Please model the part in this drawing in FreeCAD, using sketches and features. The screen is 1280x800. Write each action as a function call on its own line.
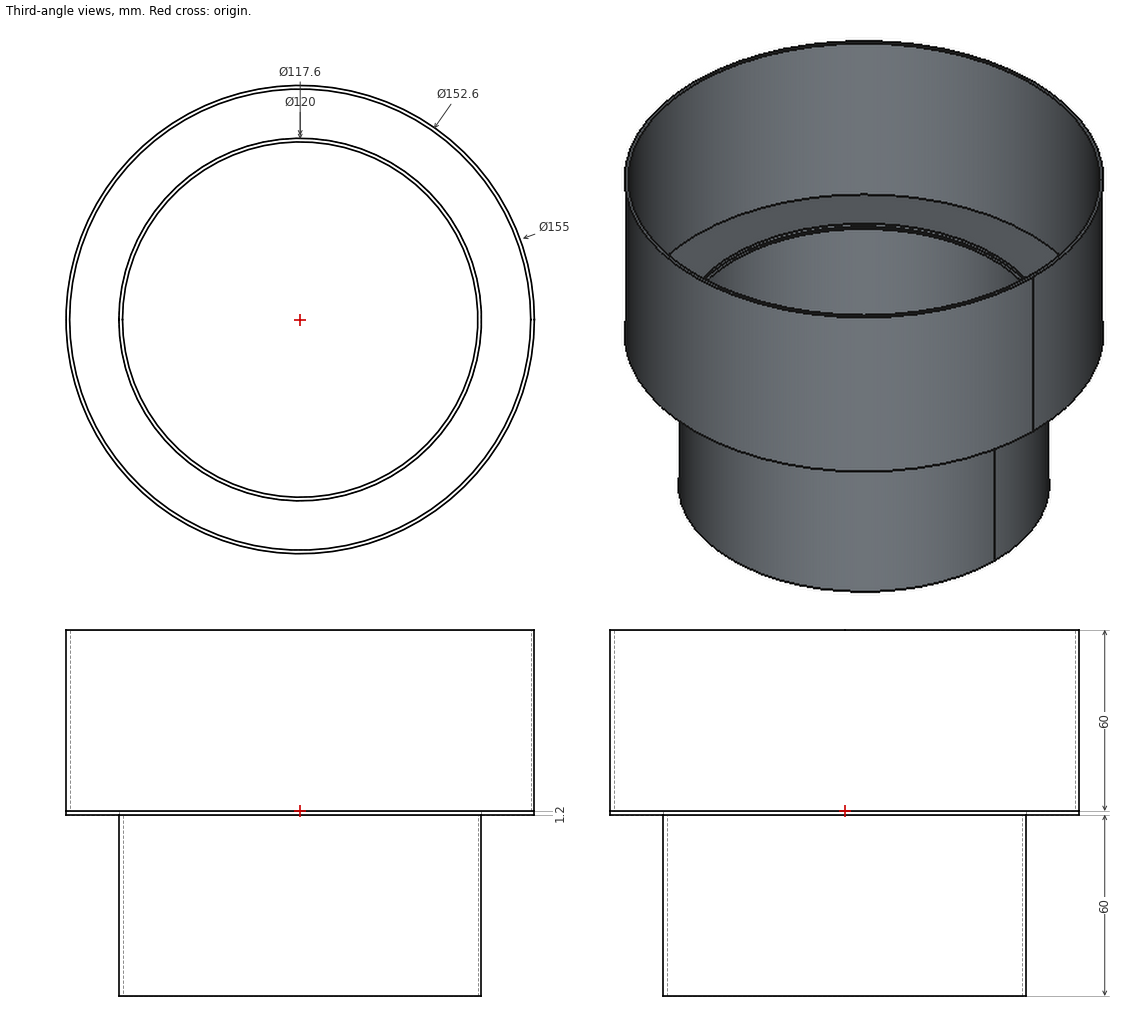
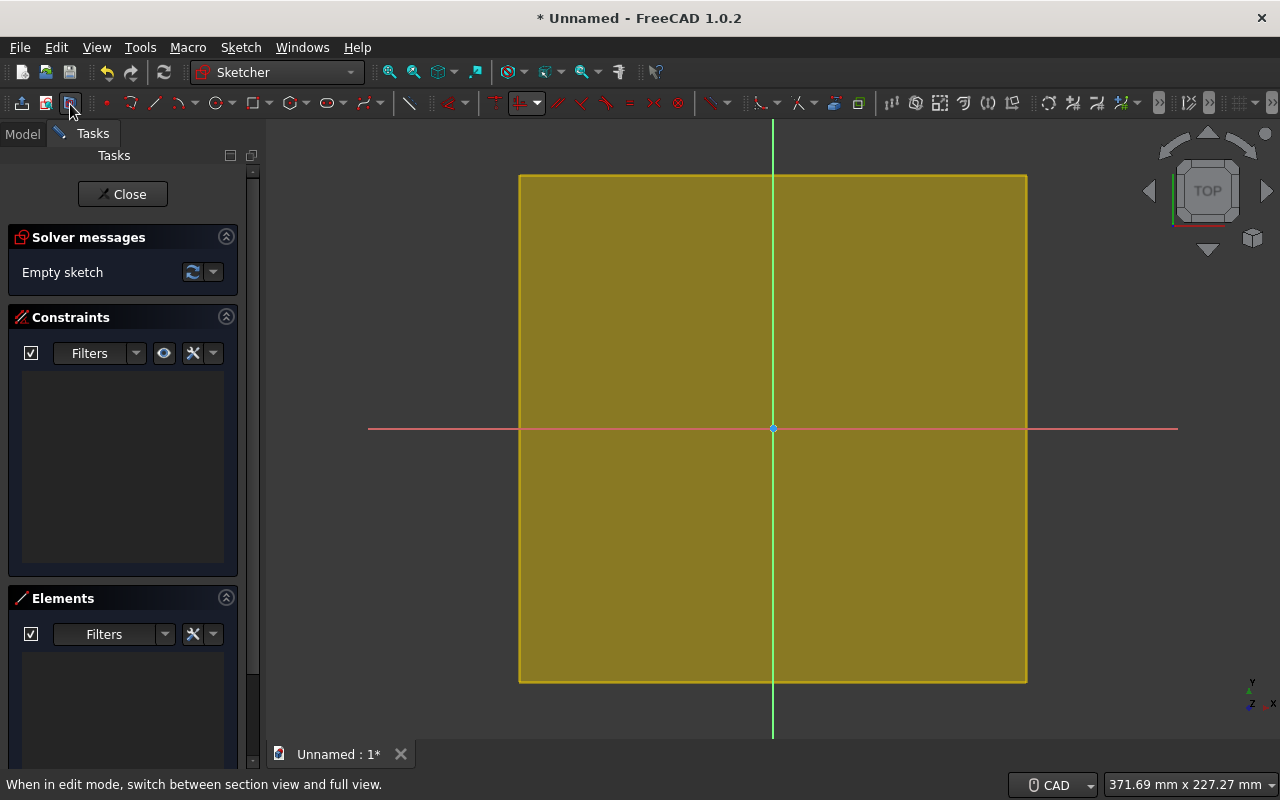
click(216, 104)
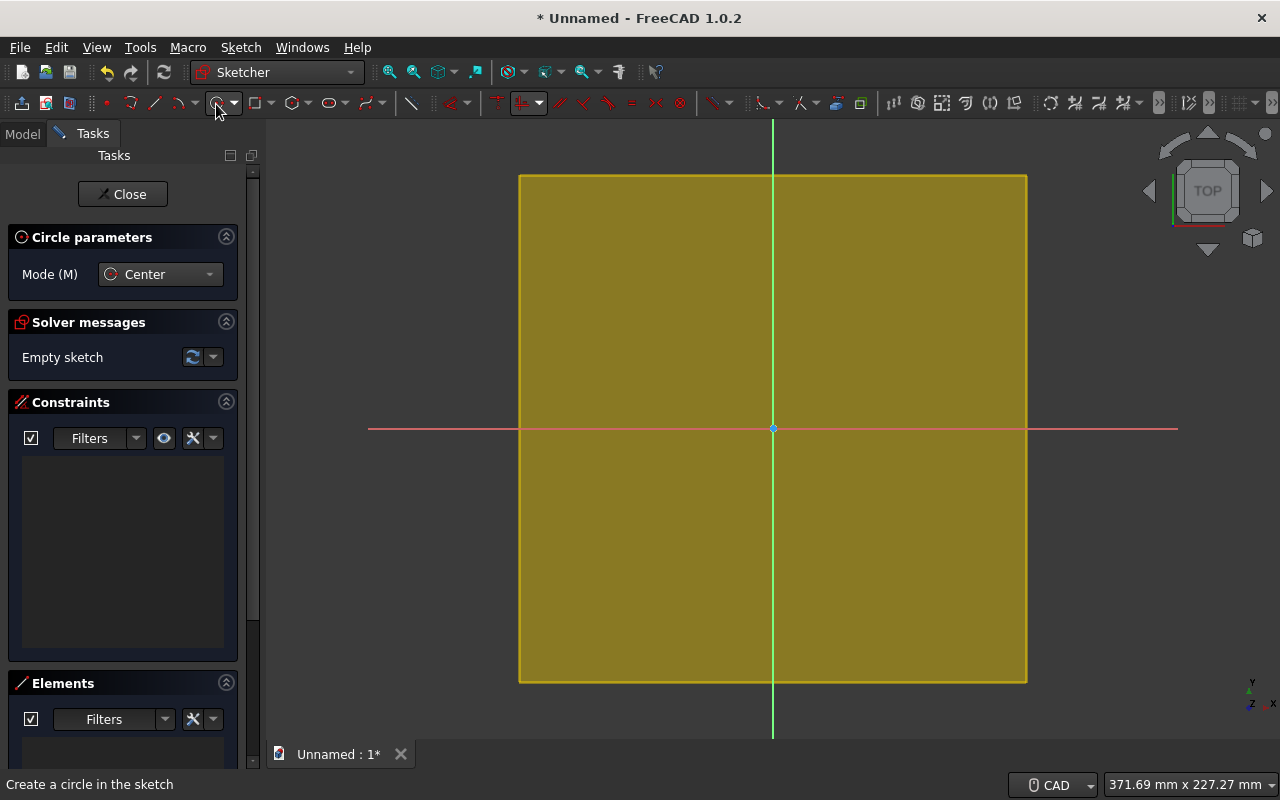
click(773, 429)
click(923, 279)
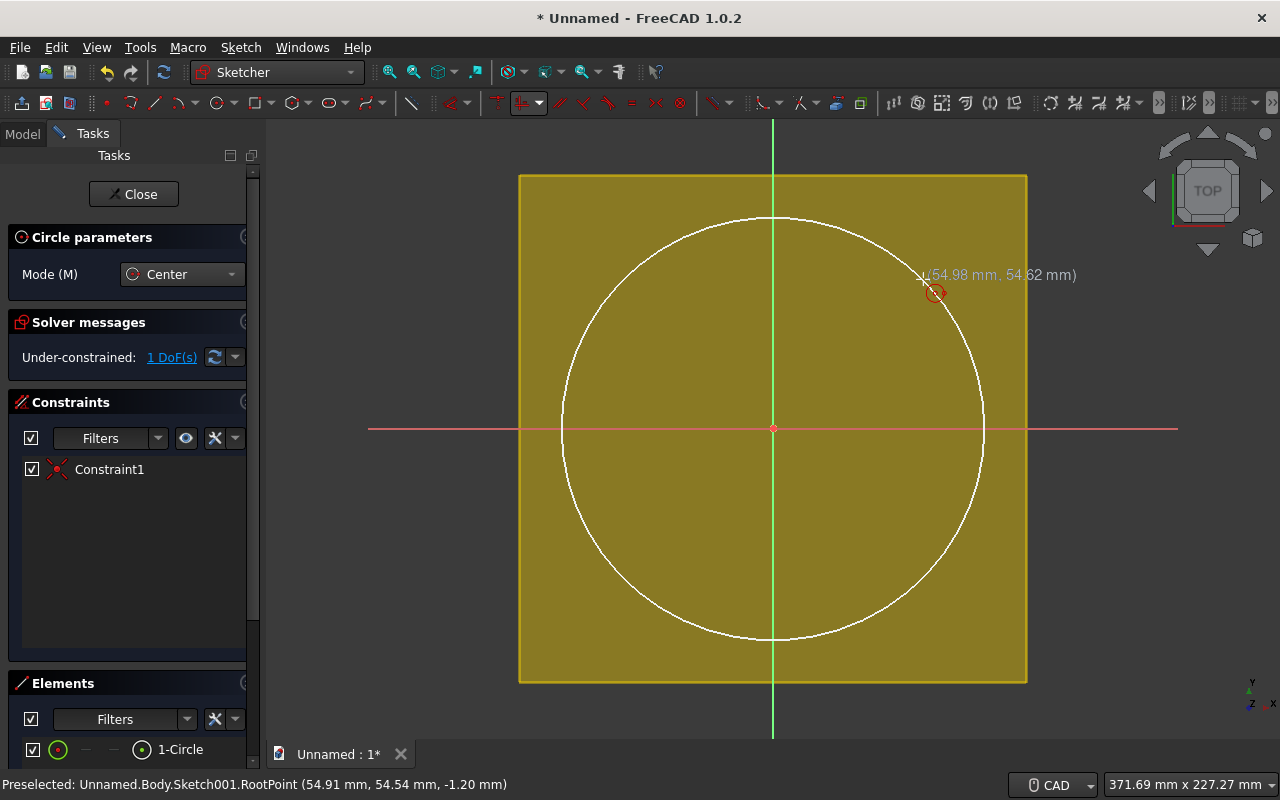
click(773, 429)
click(889, 313)
key(Escape)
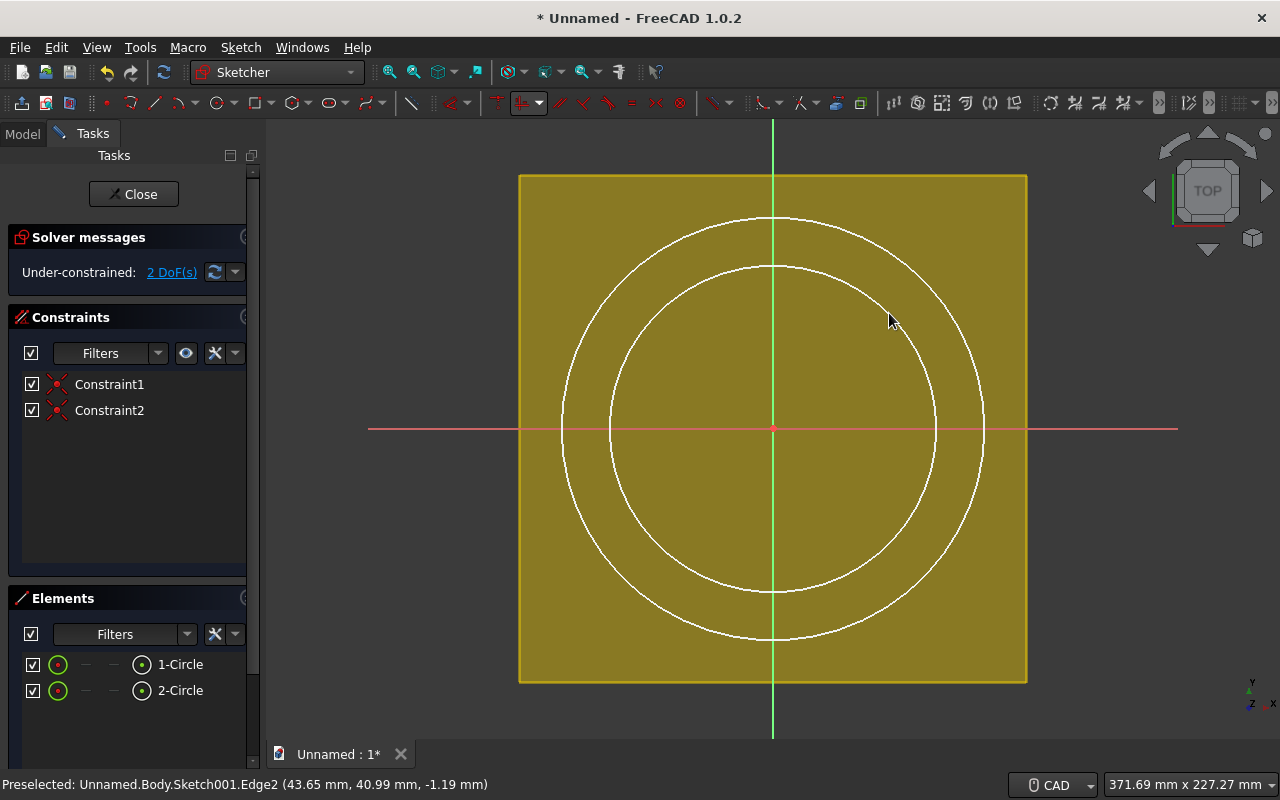
click(450, 104)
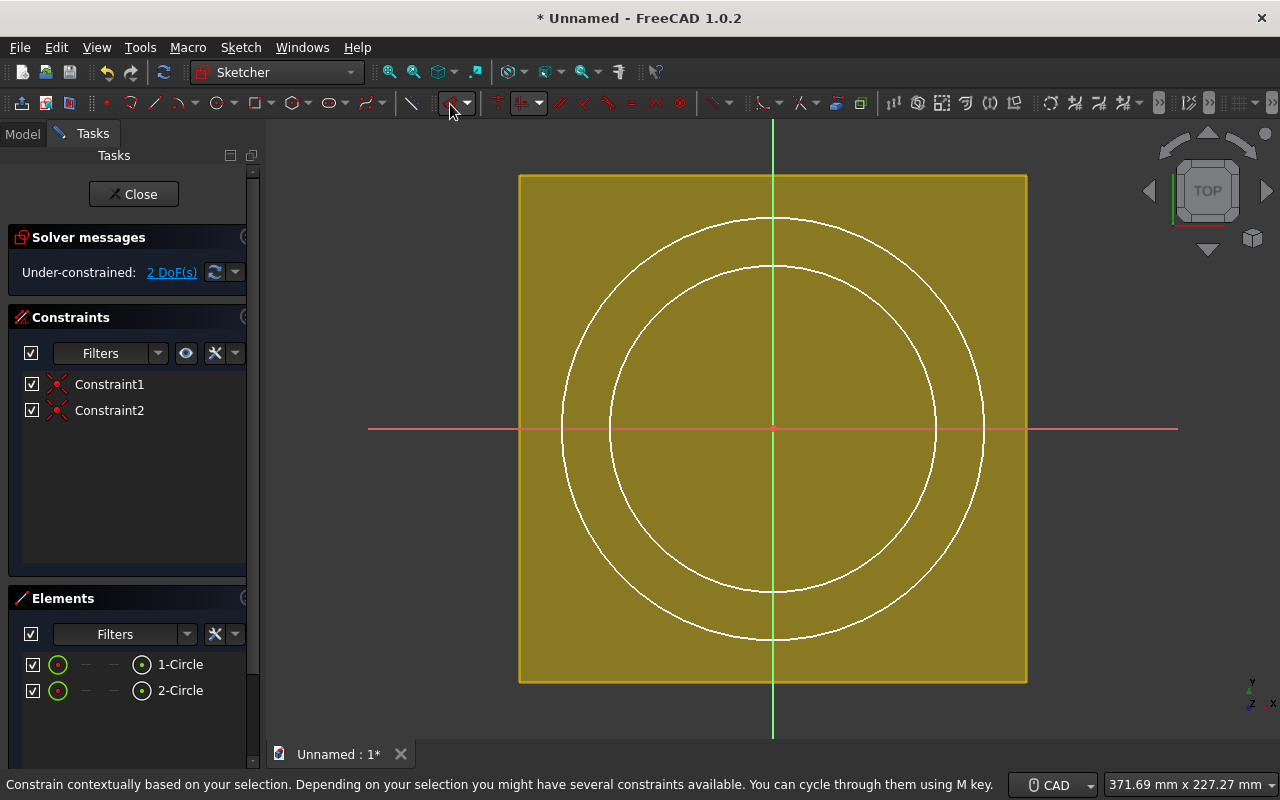
click(922, 279)
click(945, 256)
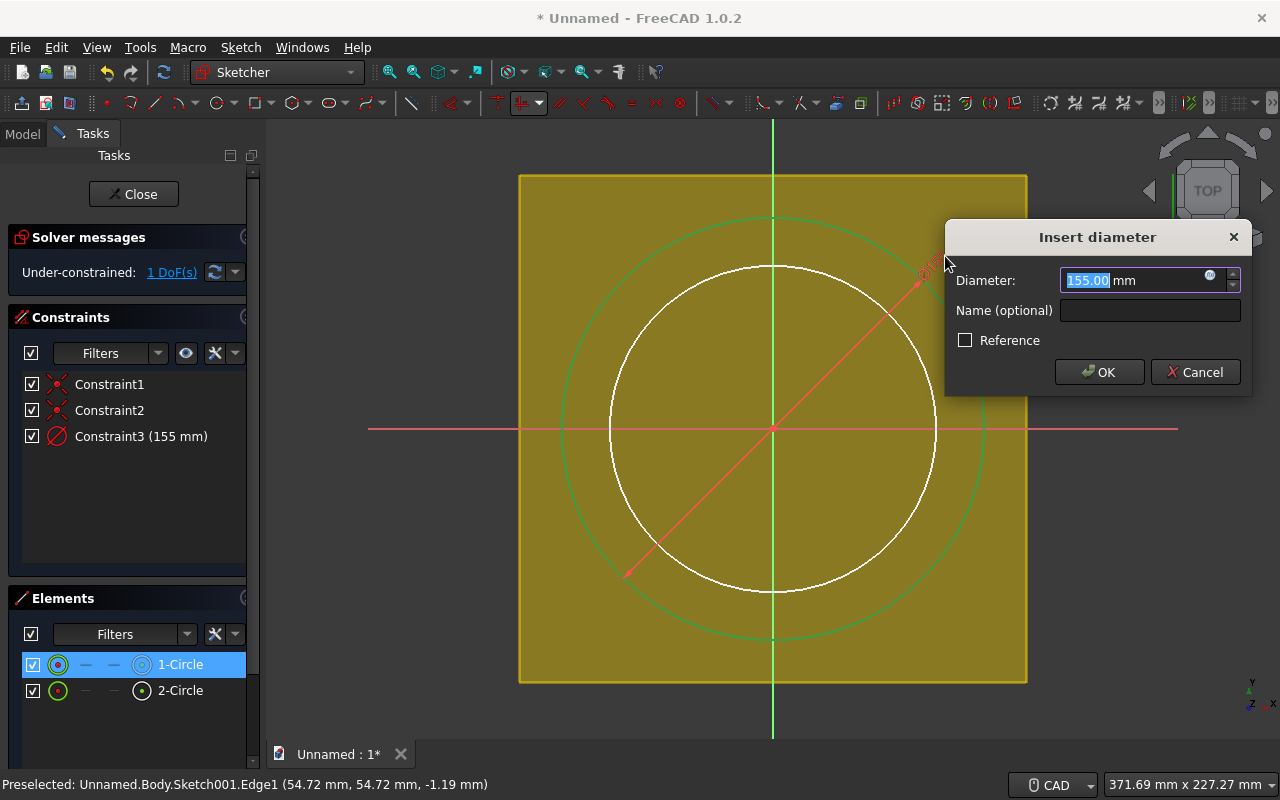
text(155)
key(Return)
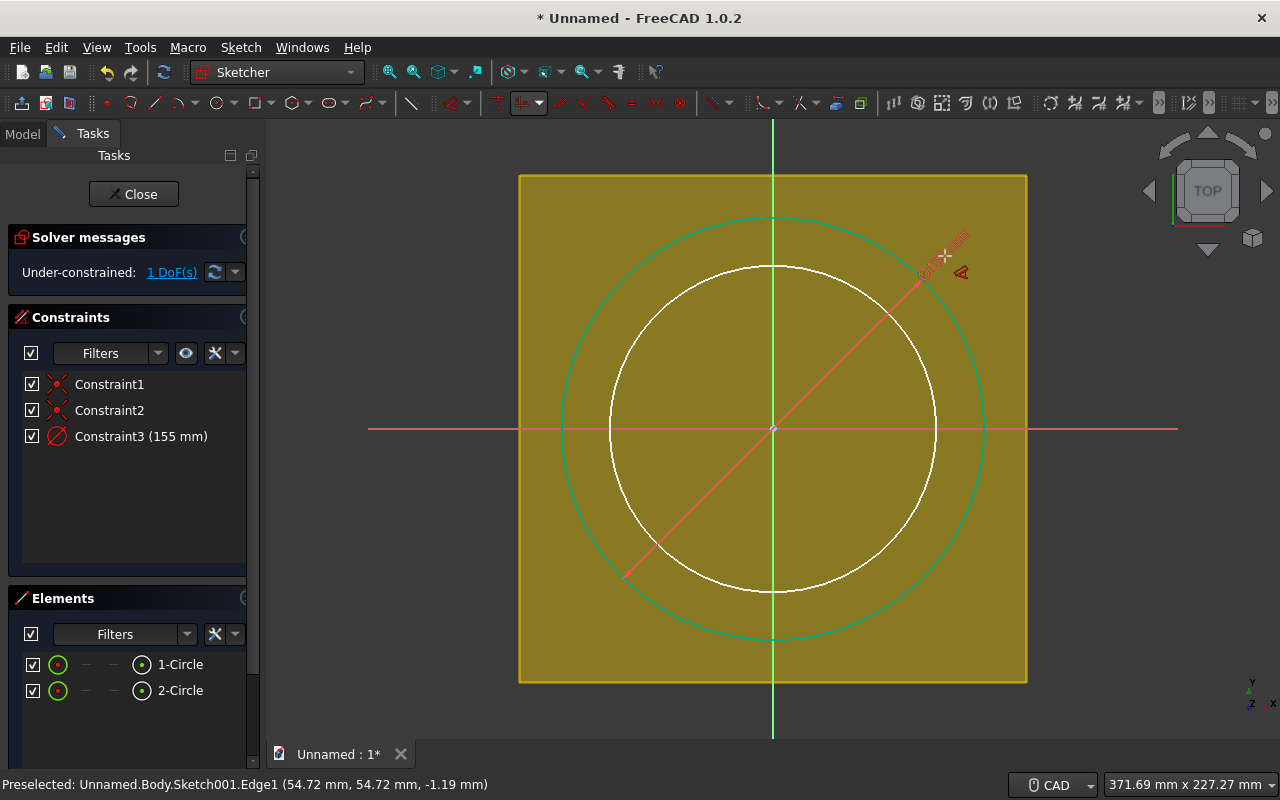
click(888, 313)
click(911, 290)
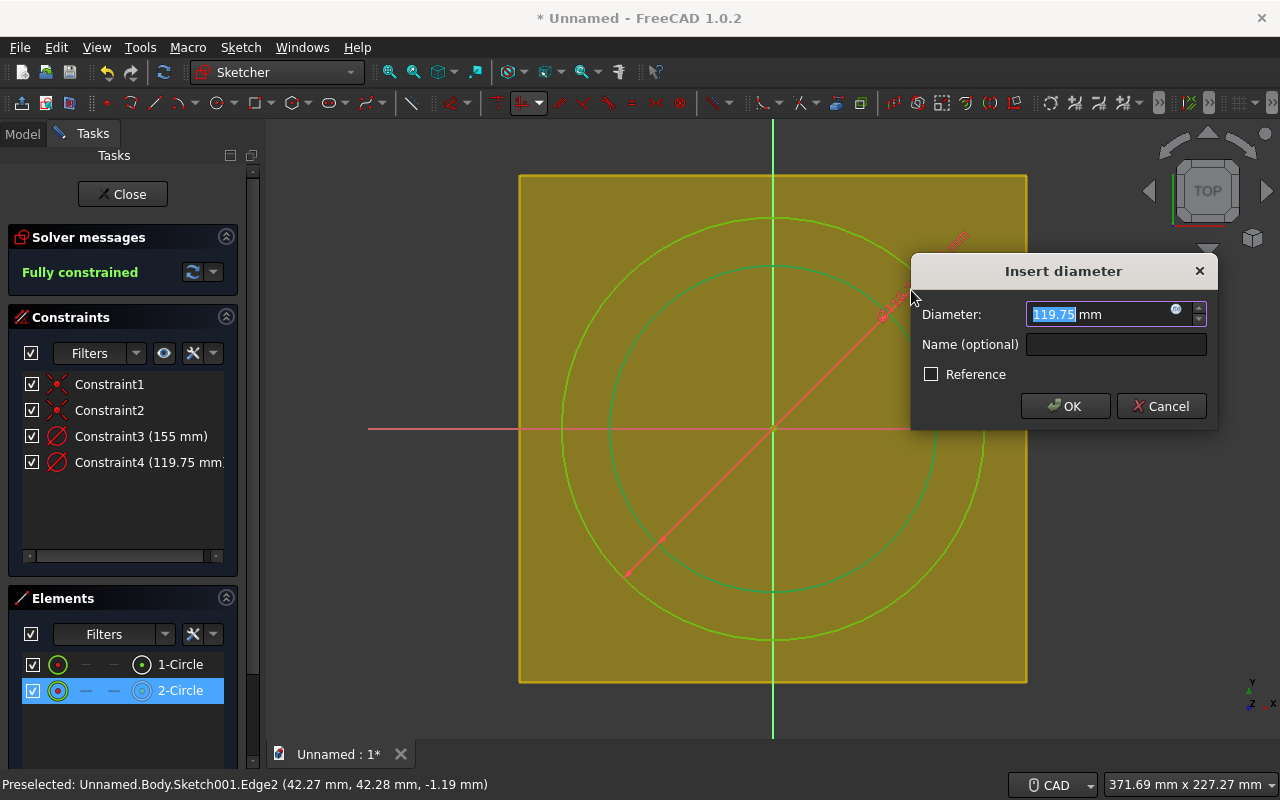
text(120)
key(Return)
key(Escape)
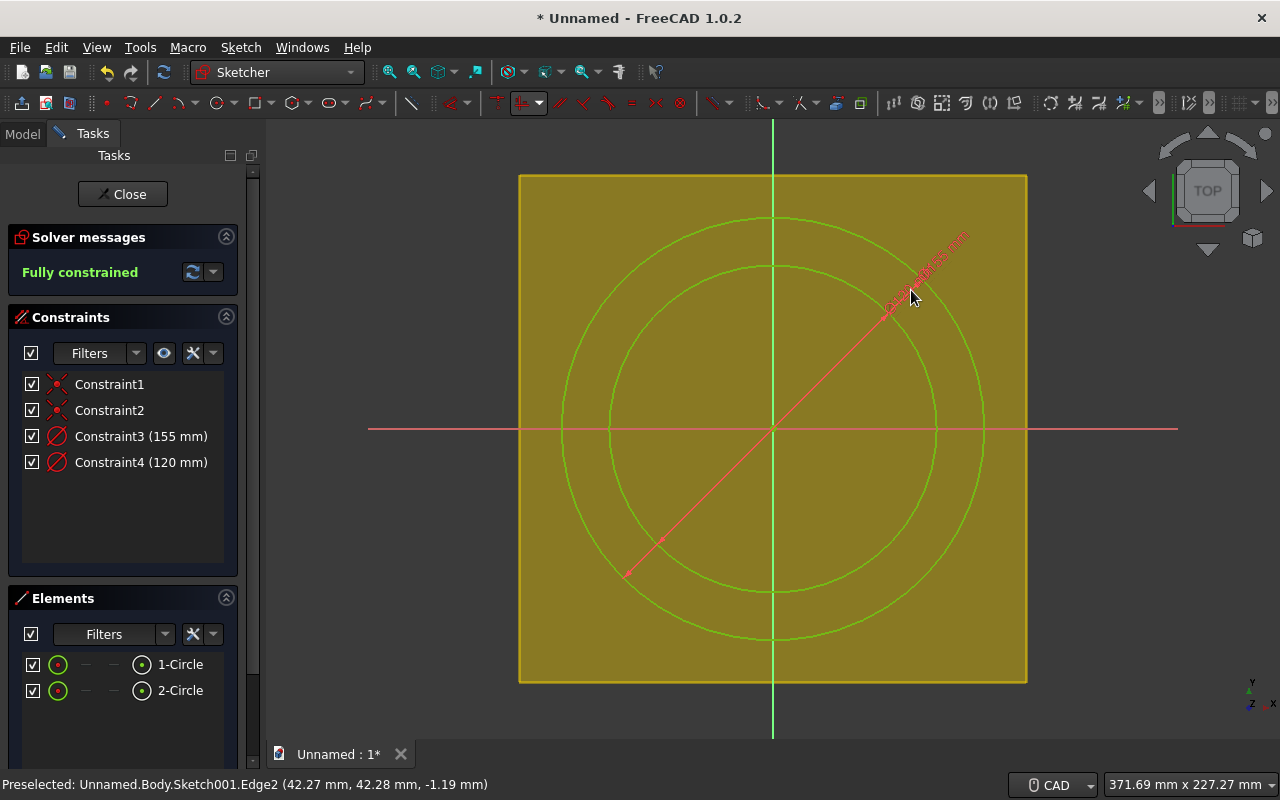
click(123, 194)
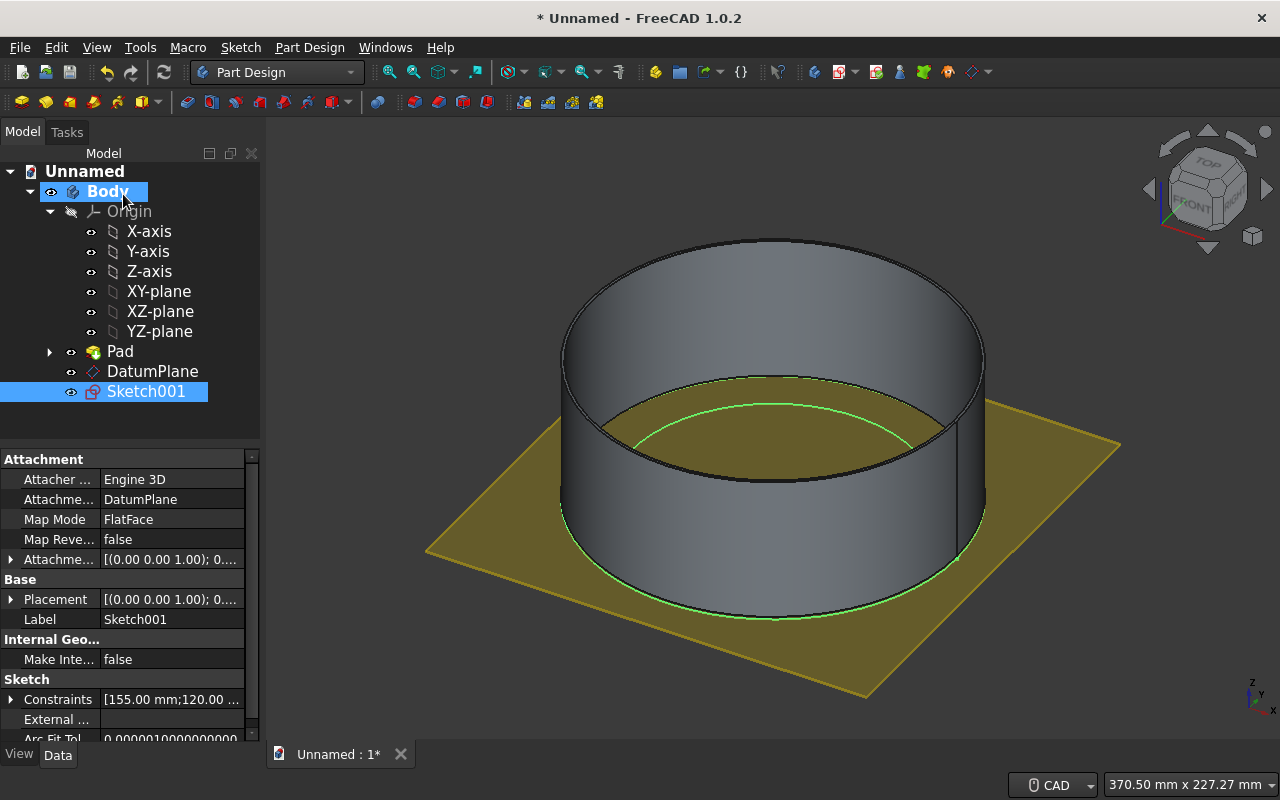
click(22, 102)